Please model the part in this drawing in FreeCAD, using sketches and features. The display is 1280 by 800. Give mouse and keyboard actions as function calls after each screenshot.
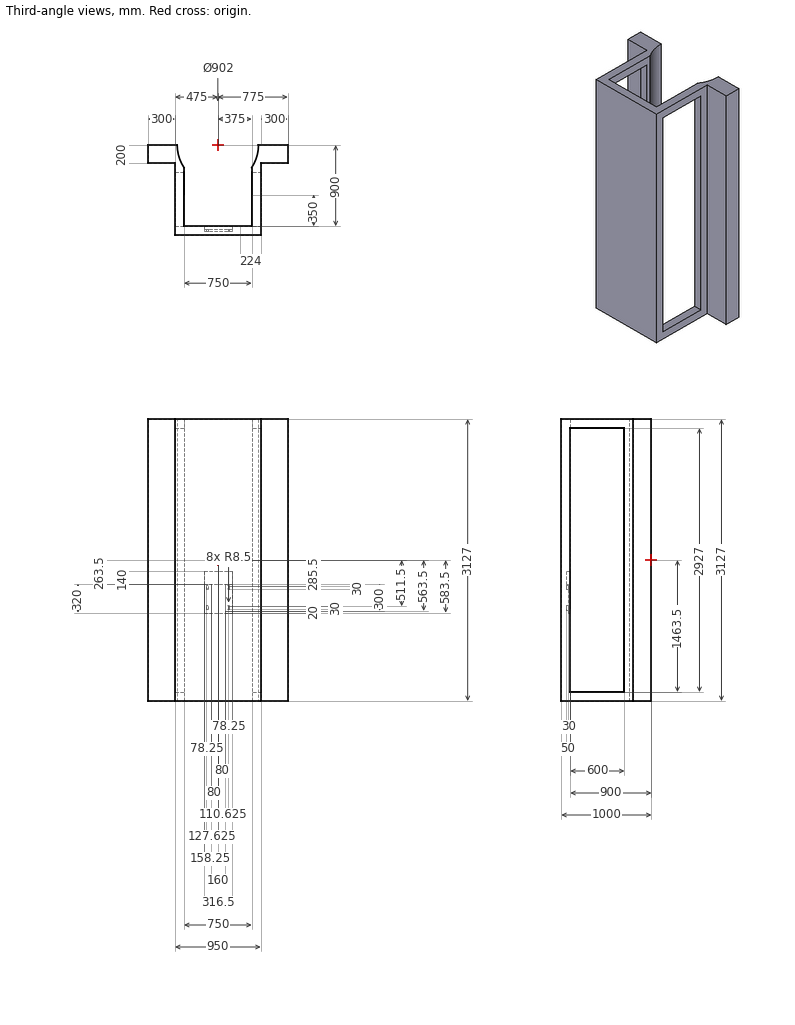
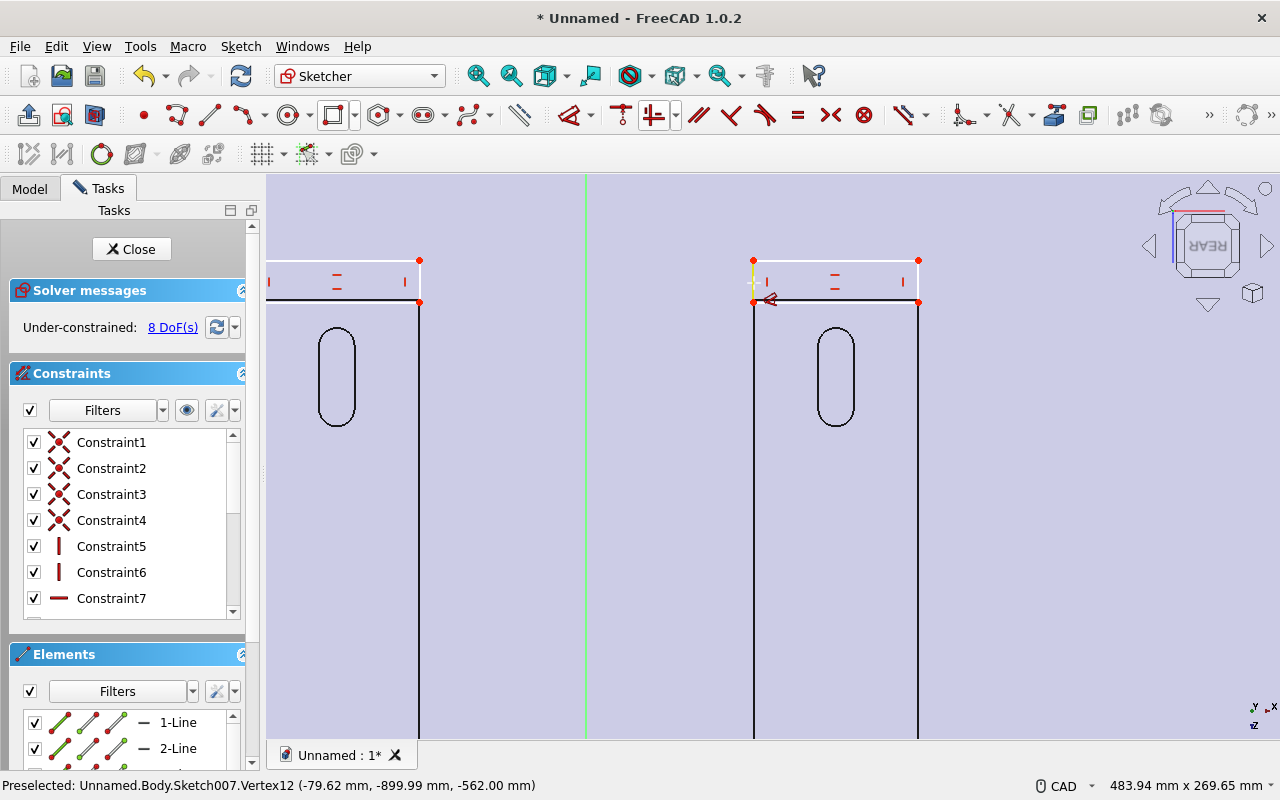
click(753, 282)
click(787, 282)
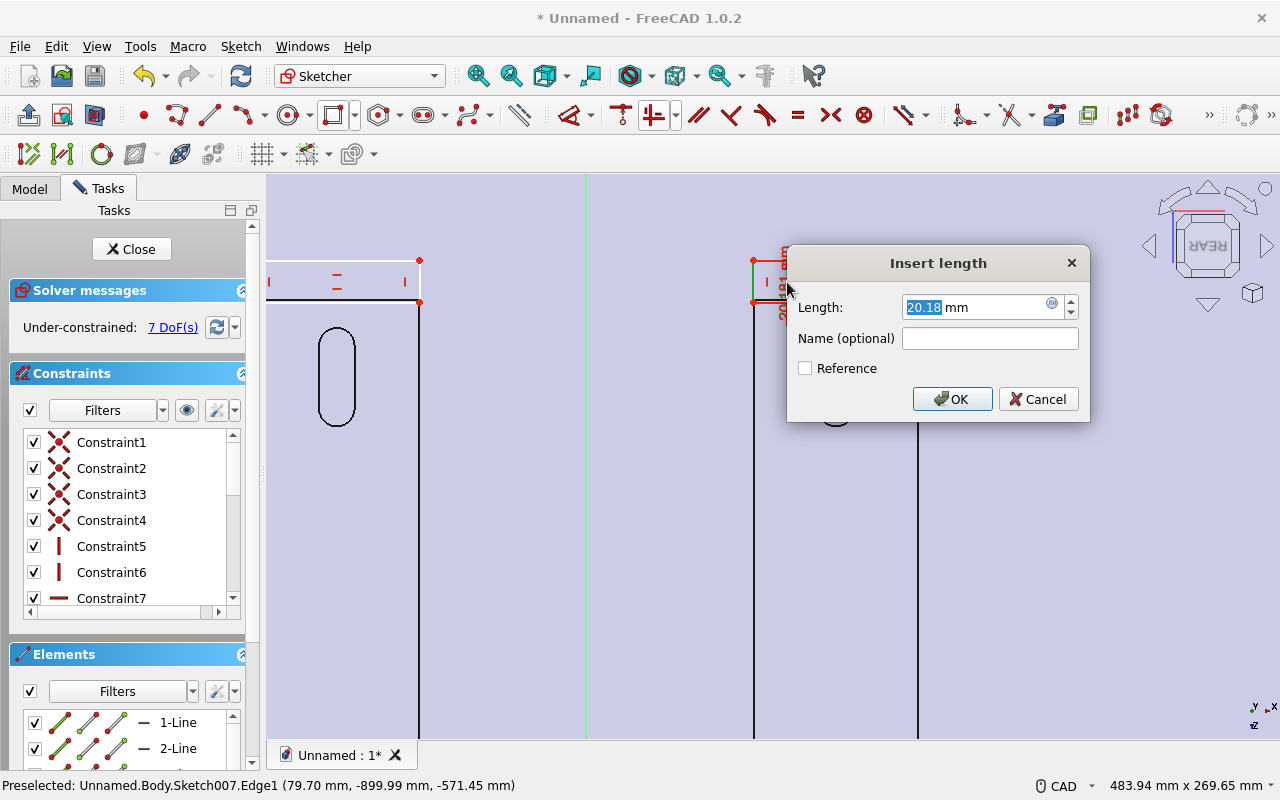
text(20)
key(Return)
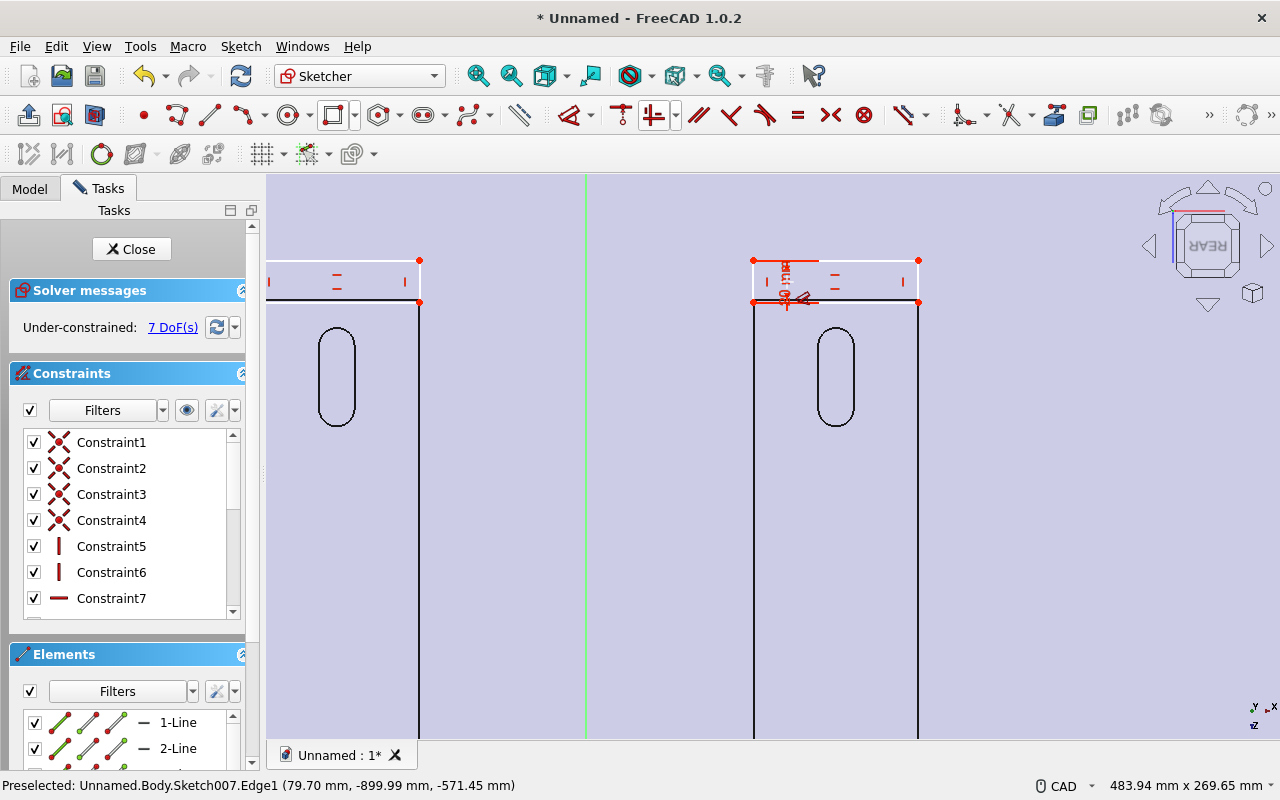
scroll(755, 279, down, 6)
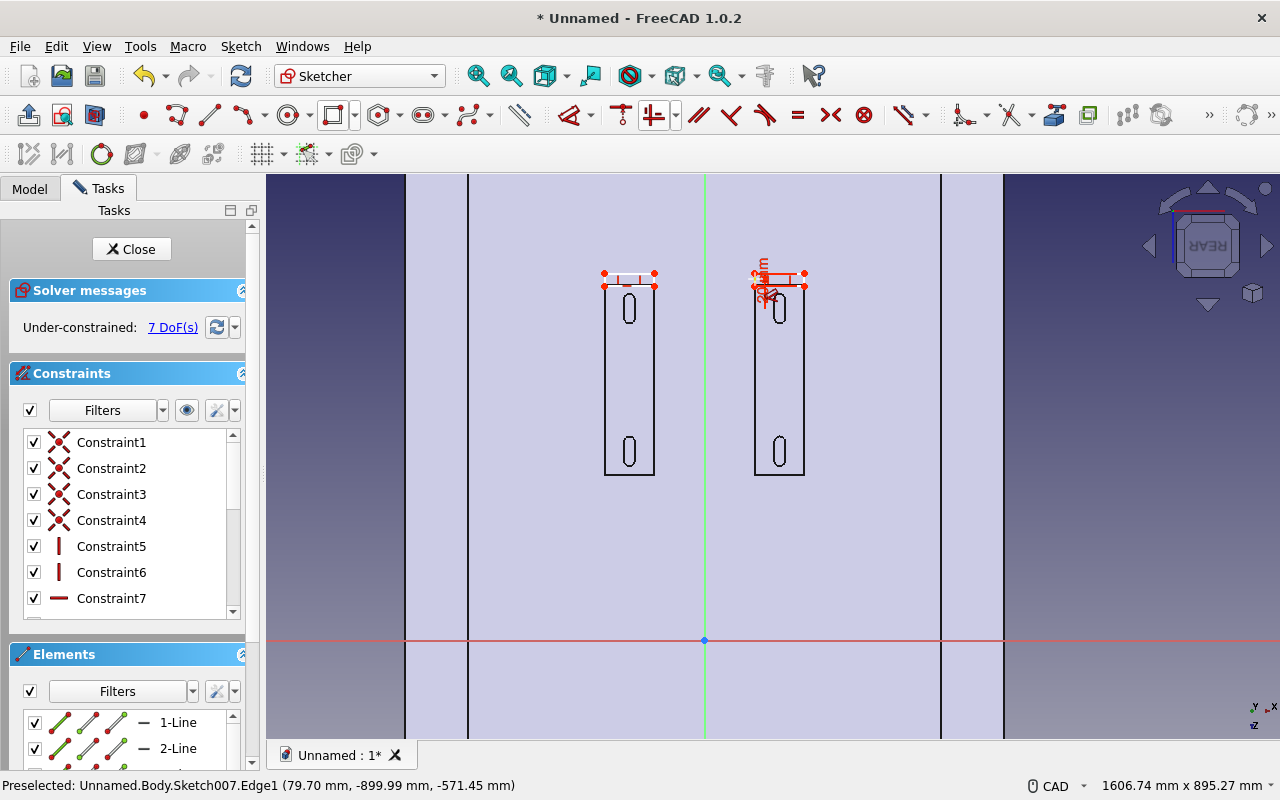
scroll(605, 277, up, 7)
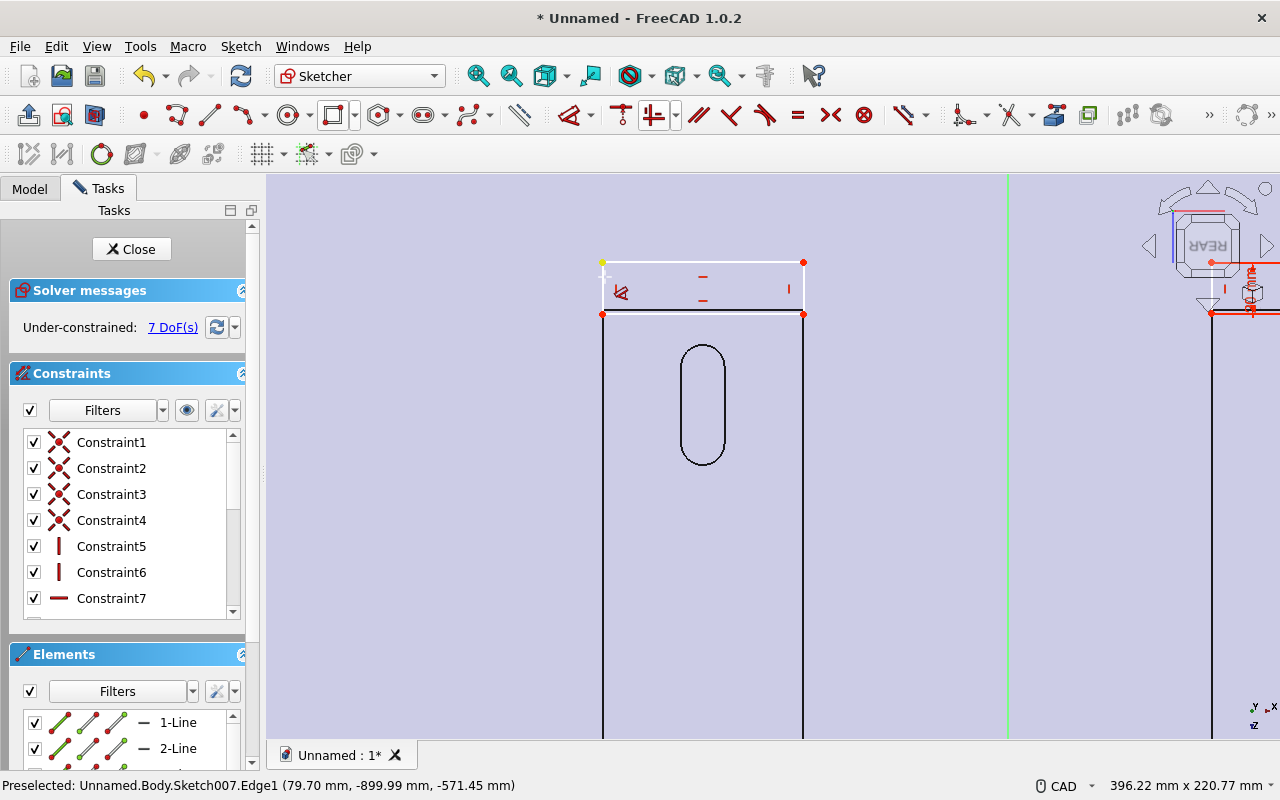
click(603, 278)
click(569, 288)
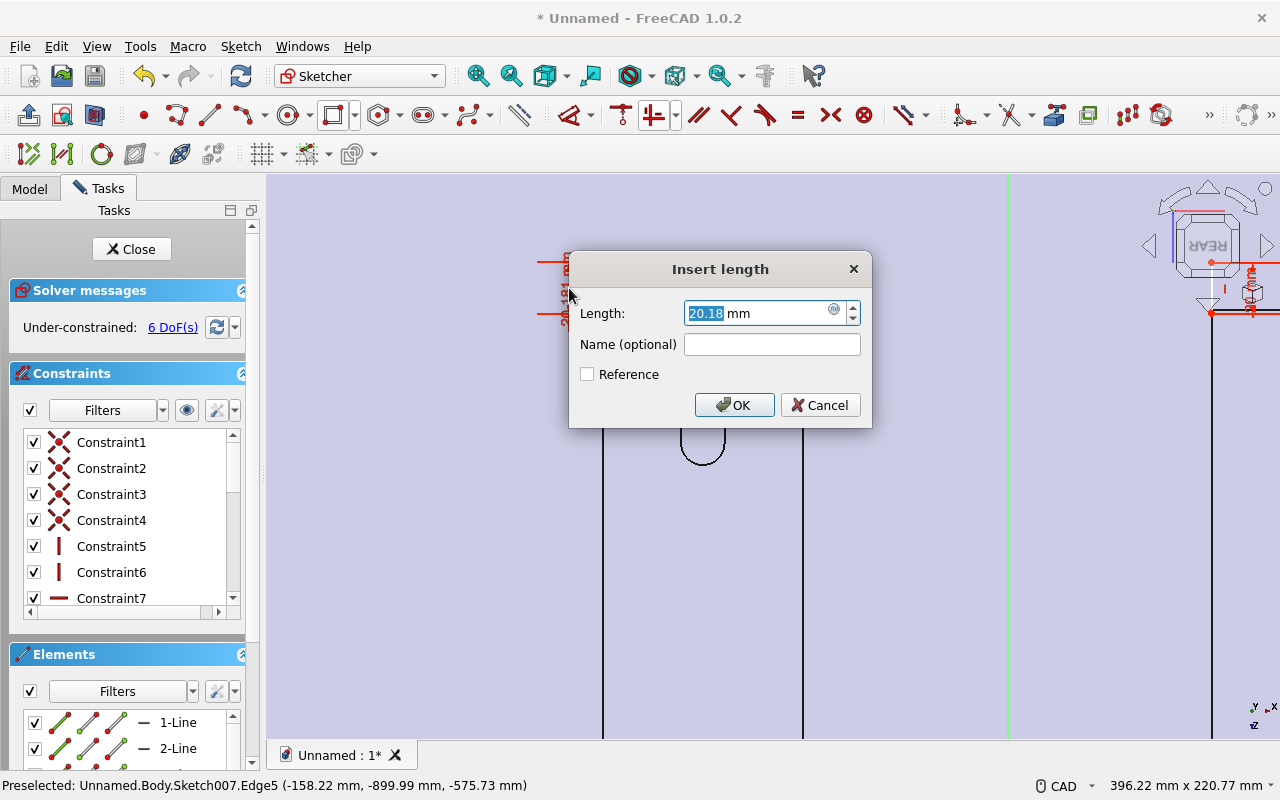
text(20)
key(Return)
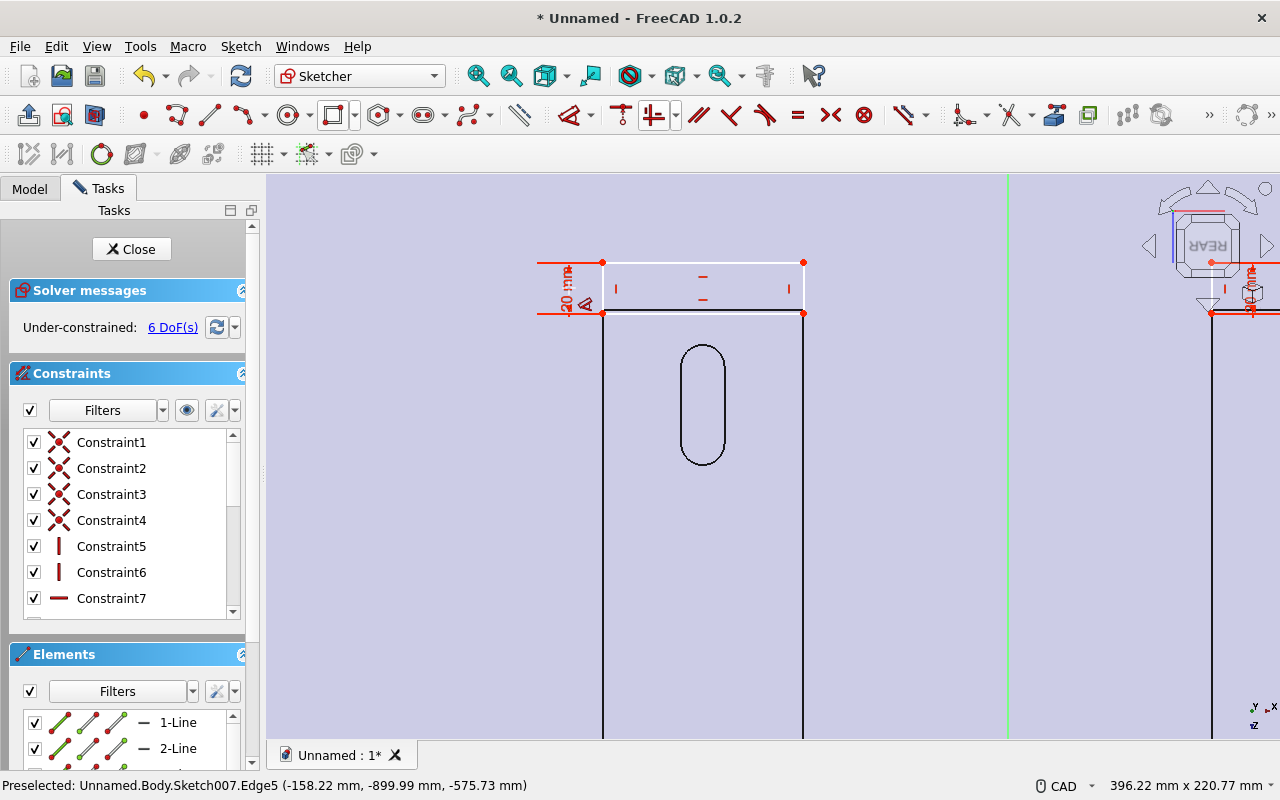
scroll(605, 277, down, 7)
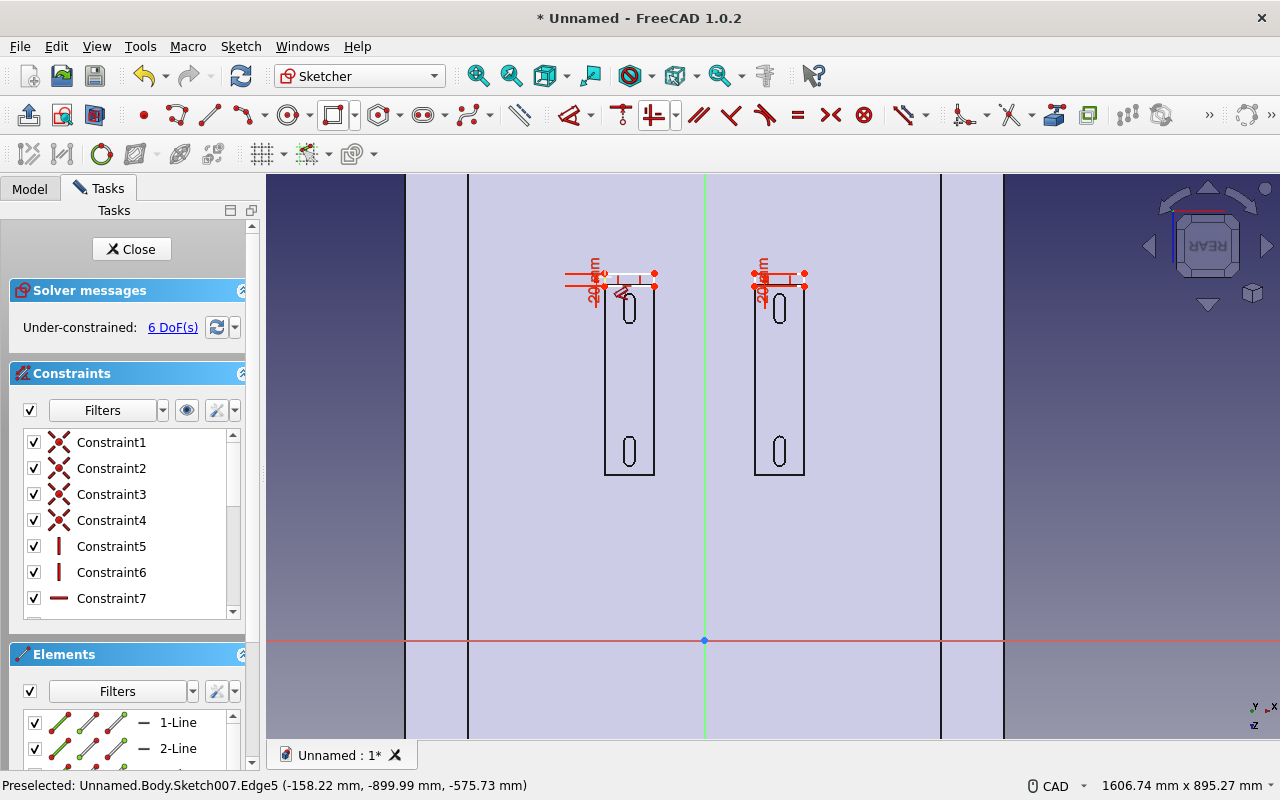
click(755, 274)
click(730, 675)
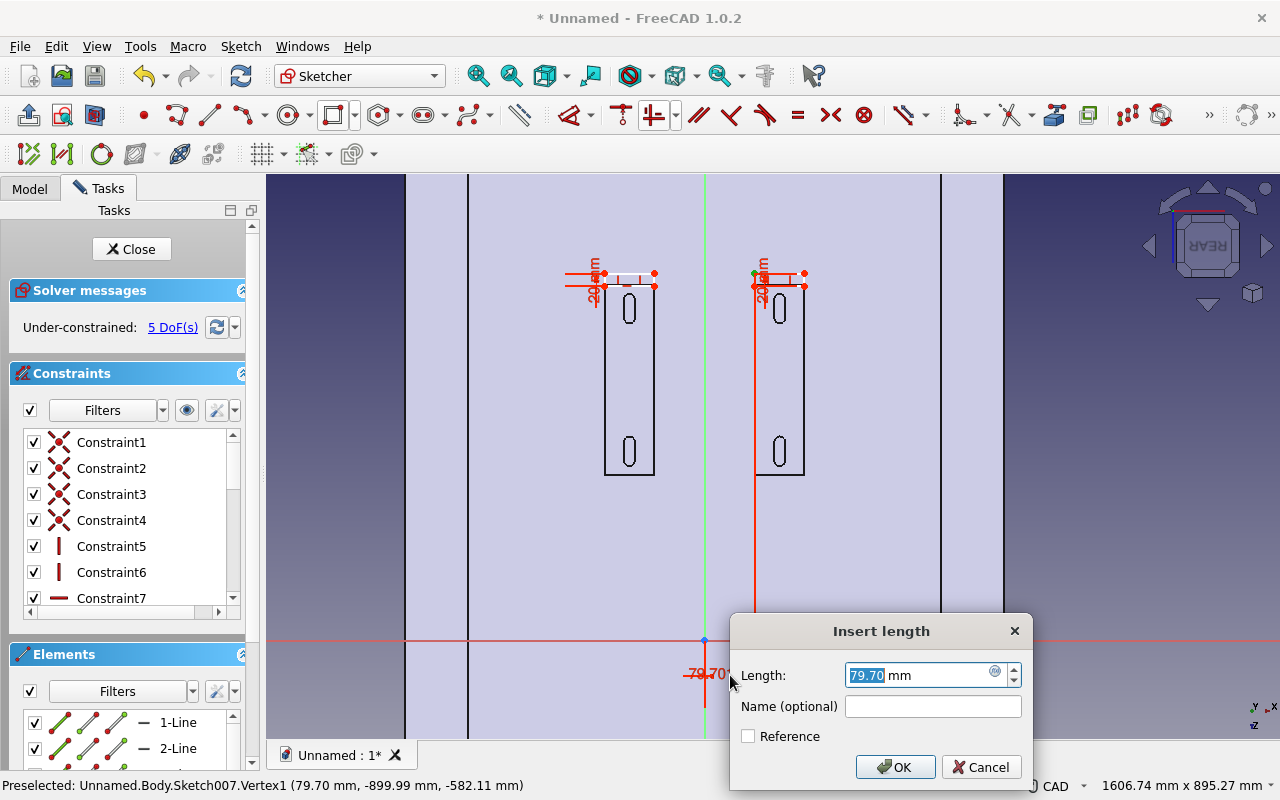
text(80)
key(Return)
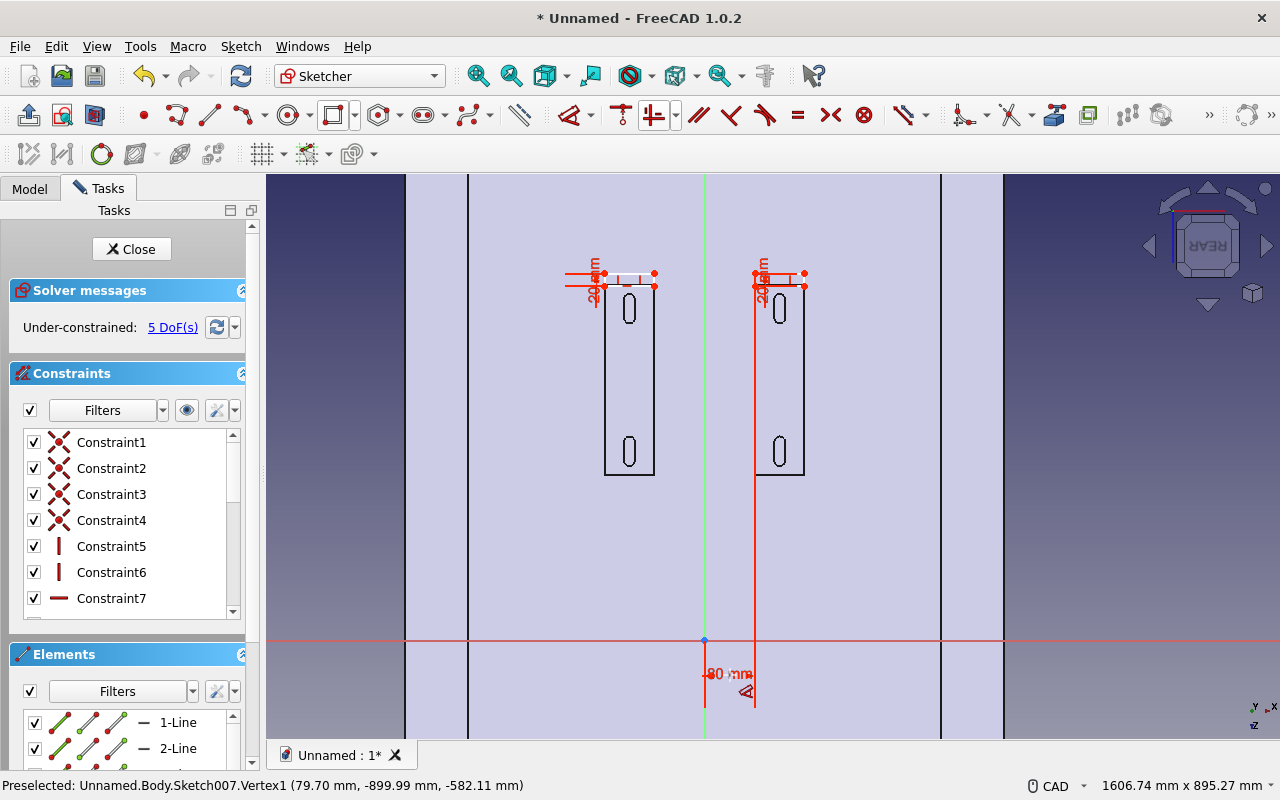
click(654, 286)
click(679, 252)